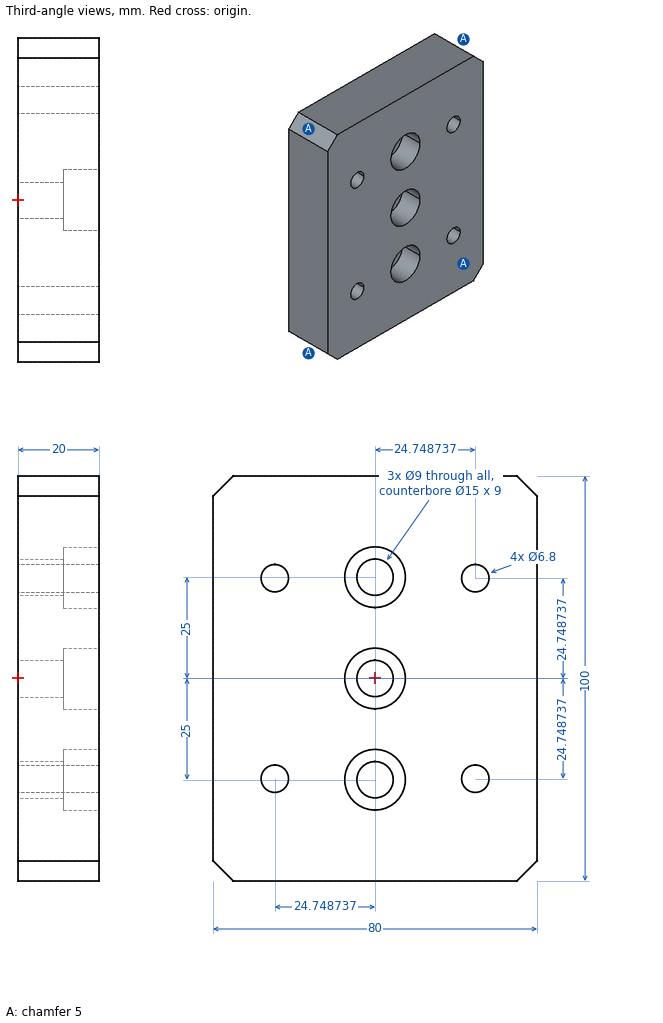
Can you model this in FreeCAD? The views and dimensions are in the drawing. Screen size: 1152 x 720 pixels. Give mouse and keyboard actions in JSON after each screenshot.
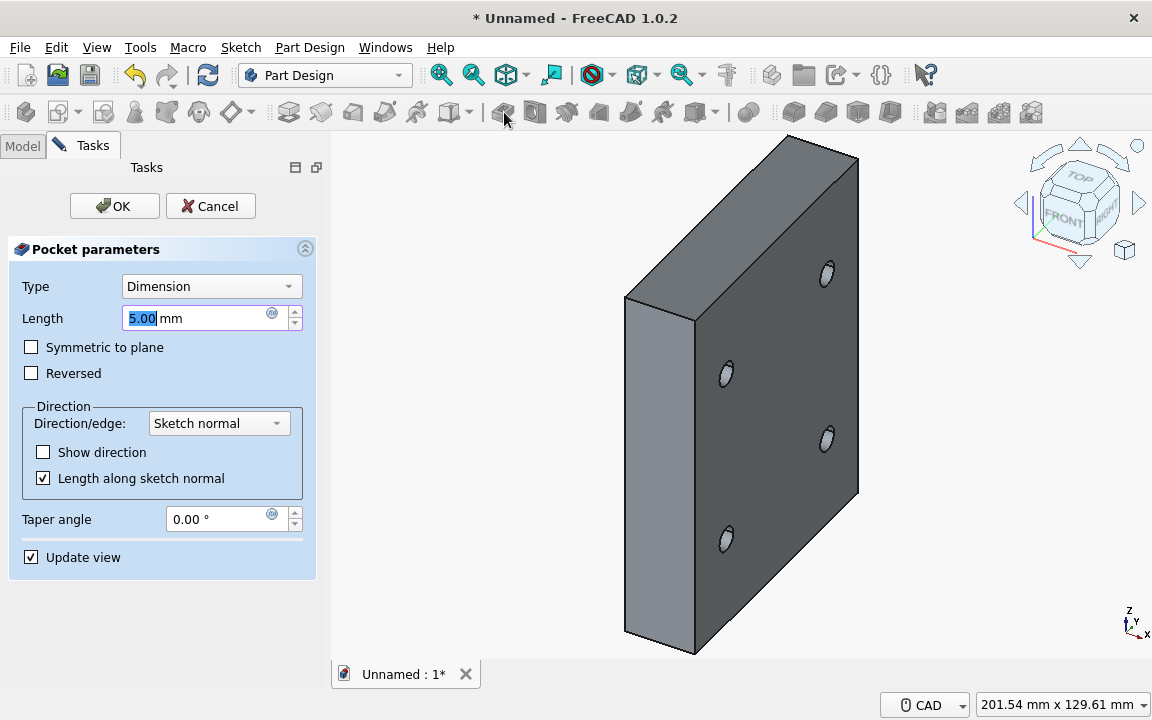
{"action": "left_click", "coordinate": [212, 286]}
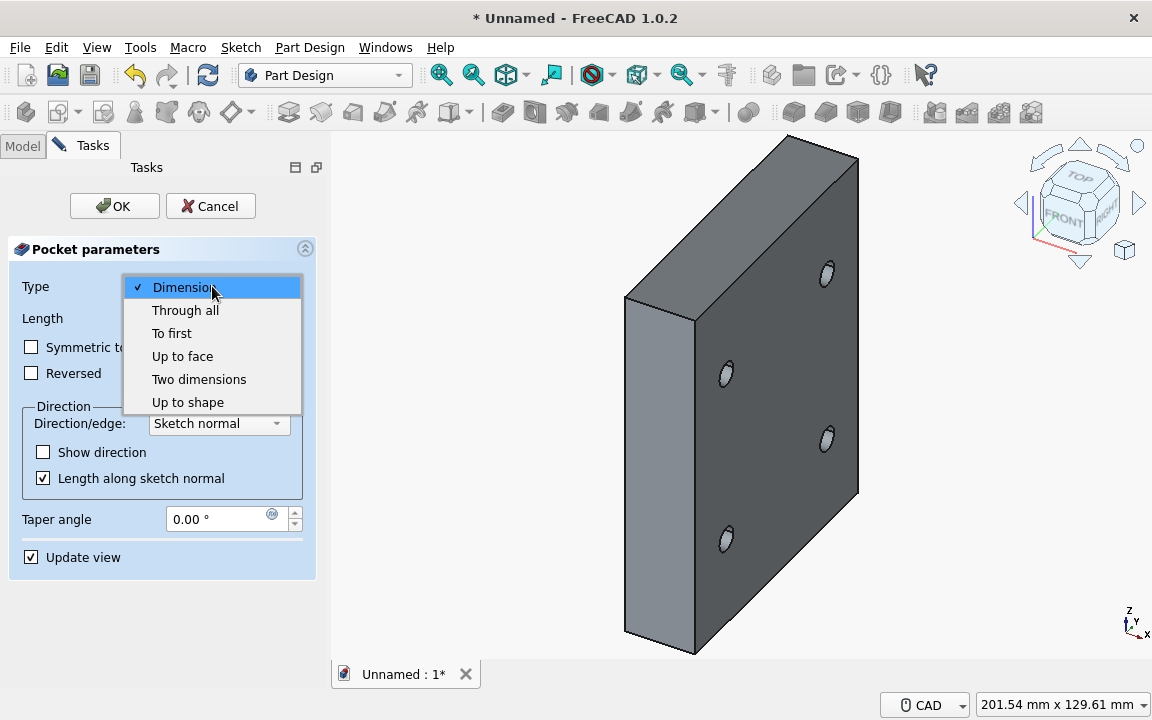
{"action": "left_click", "coordinate": [212, 310]}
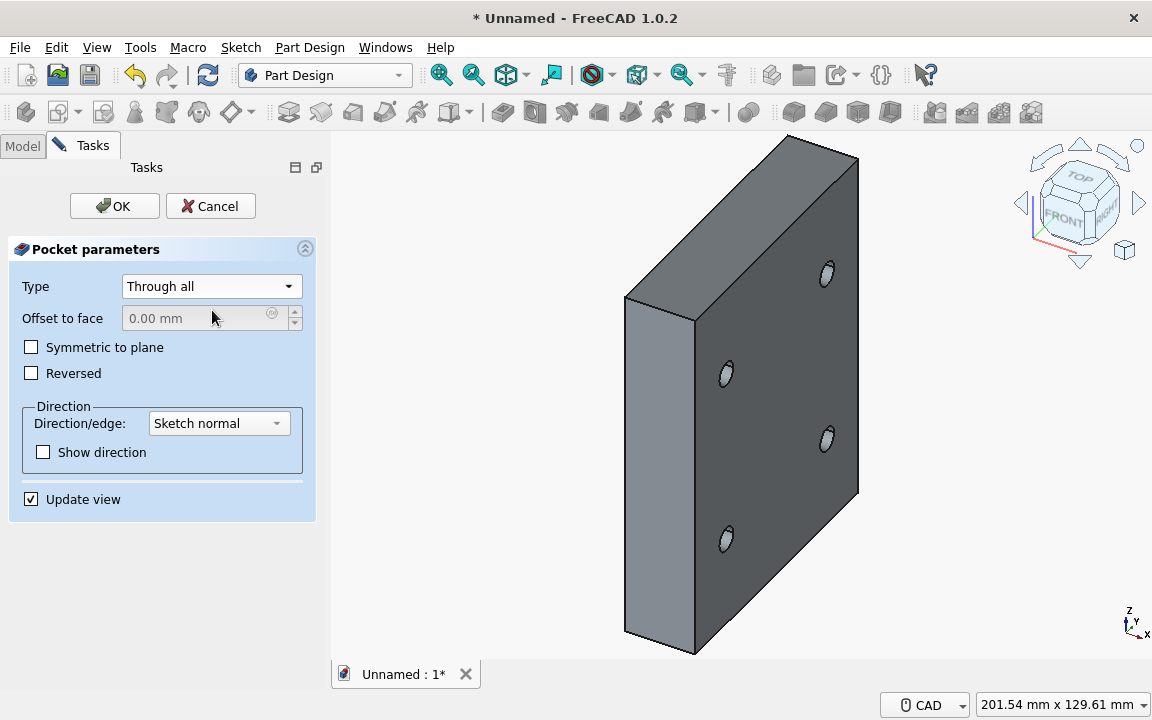
{"action": "left_click", "coordinate": [115, 206]}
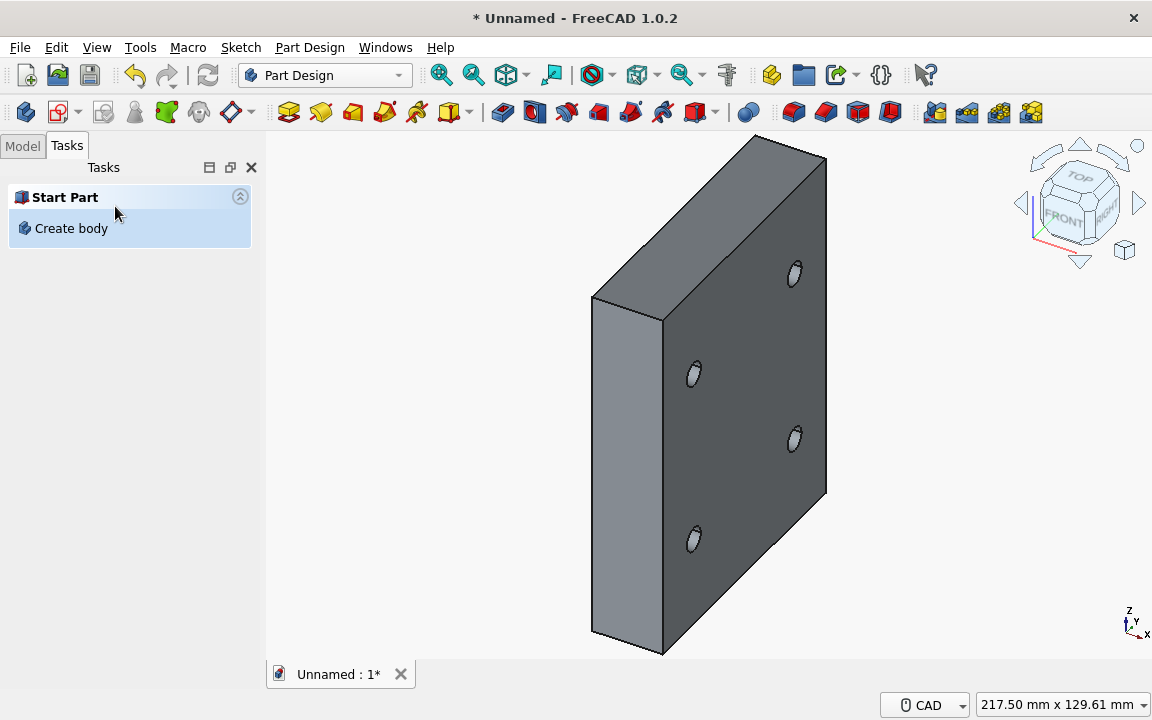
{"action": "left_click", "coordinate": [744, 406]}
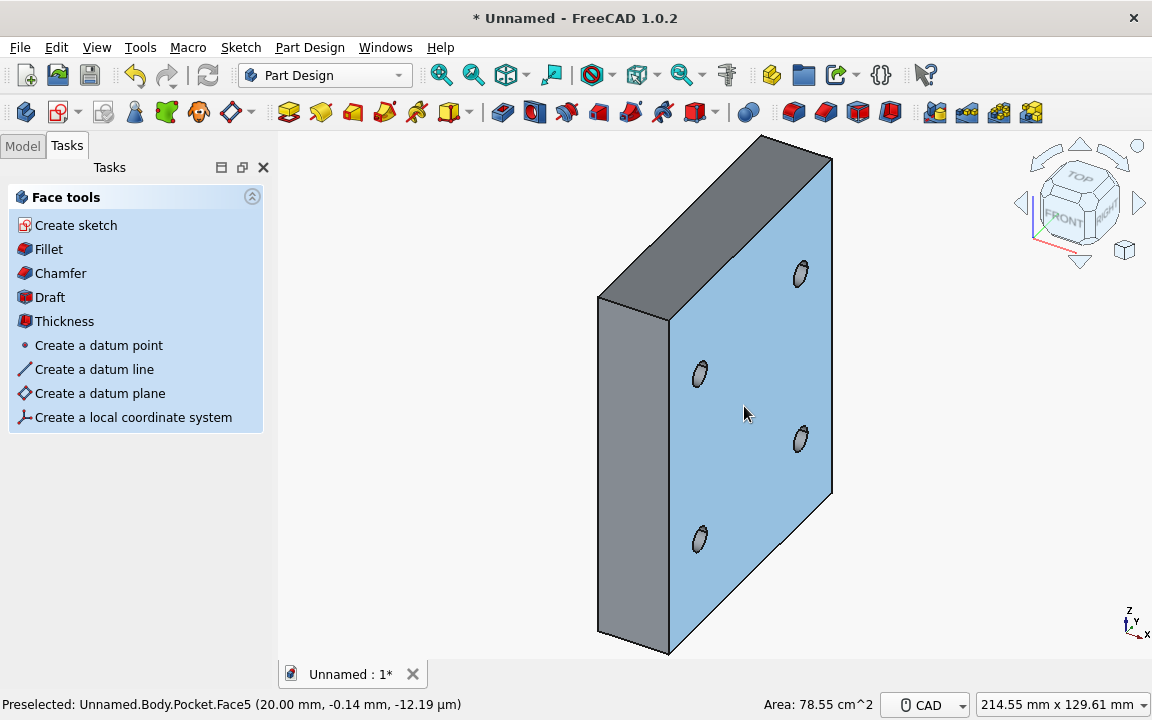
{"action": "left_click", "coordinate": [58, 112]}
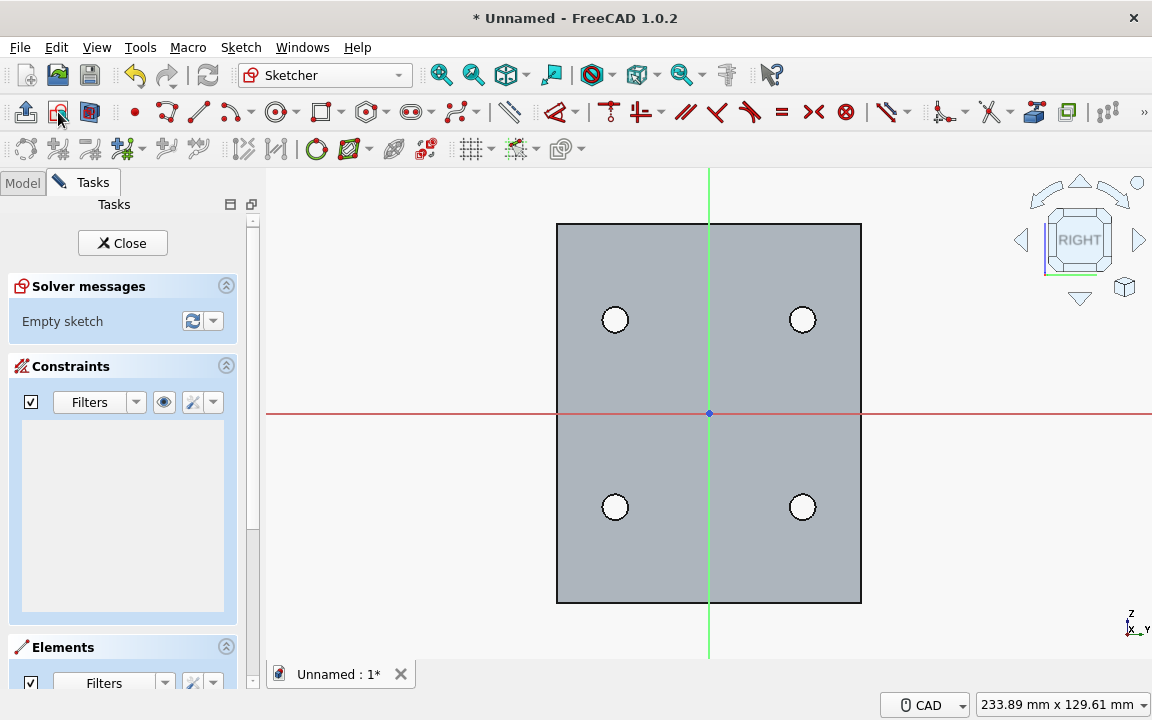
{"action": "scroll", "coordinate": [848, 413], "scroll_direction": "up", "scroll_amount": 2}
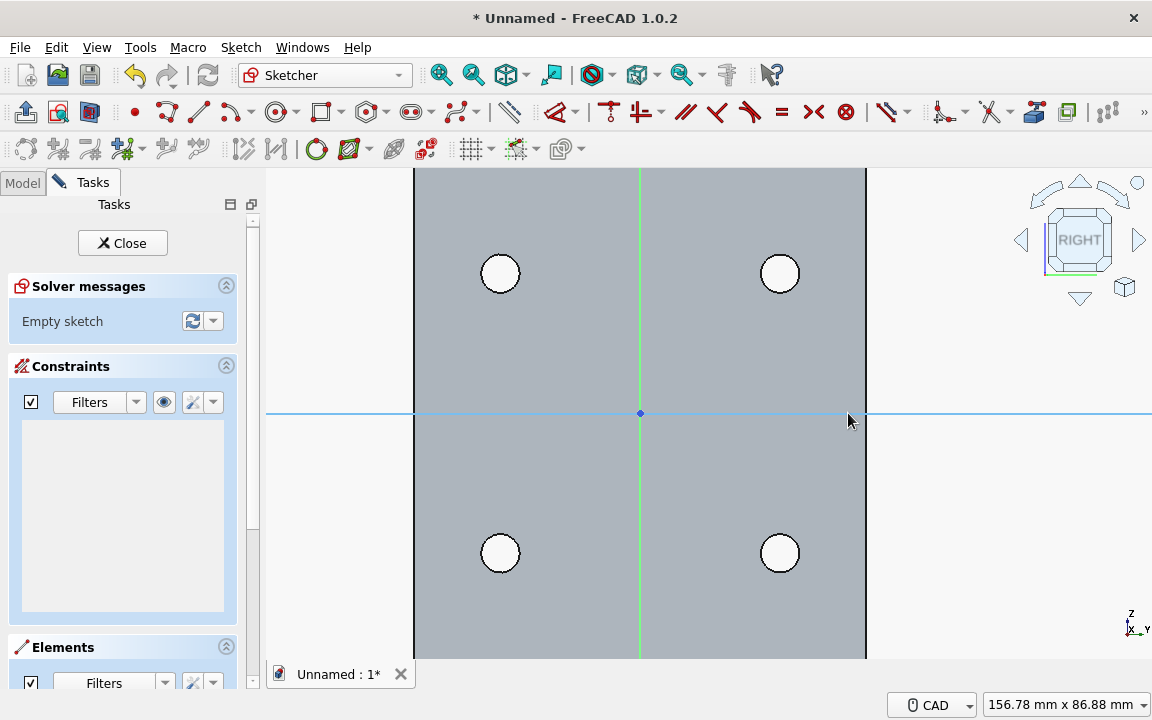
{"action": "key", "text": "g c"}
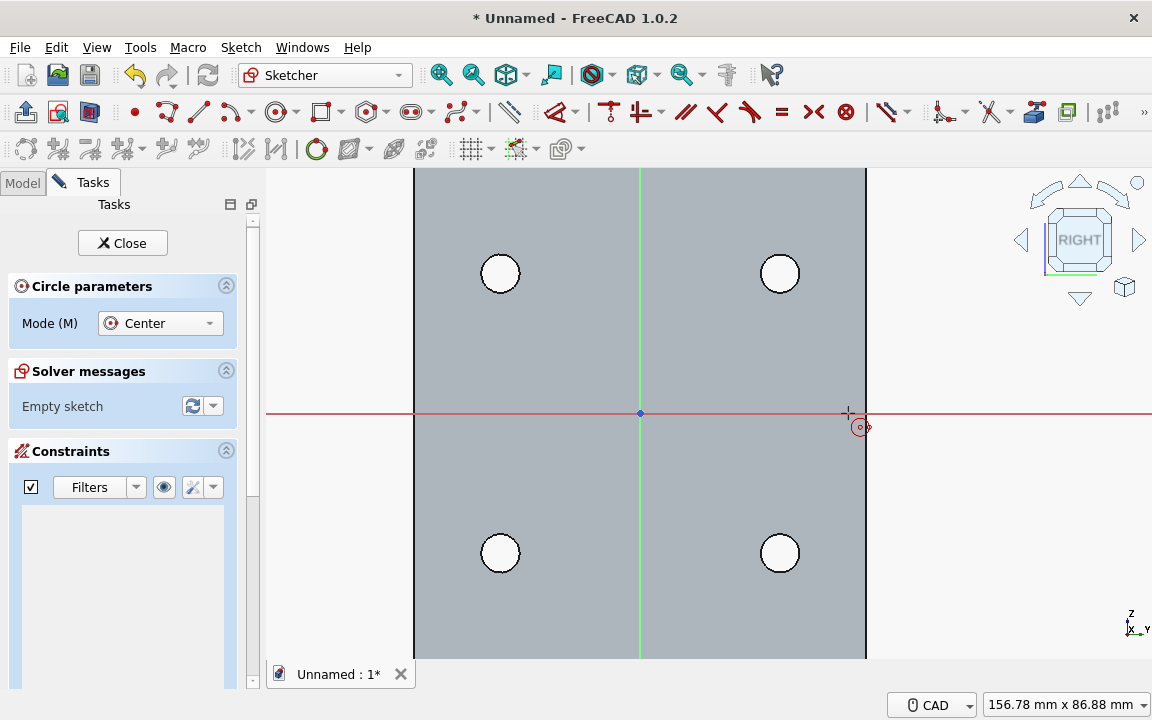
{"action": "left_click", "coordinate": [640, 272]}
{"action": "mouse_move", "coordinate": [658, 254]}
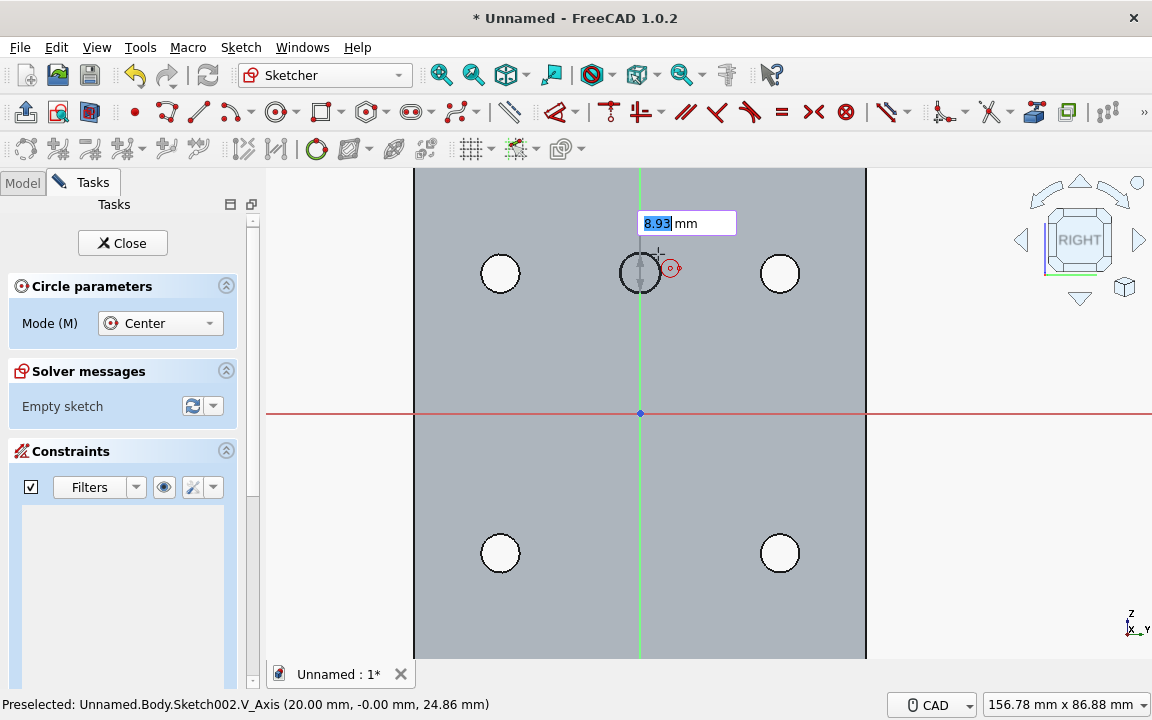
{"action": "type", "text": "9"}
{"action": "key", "text": "Return"}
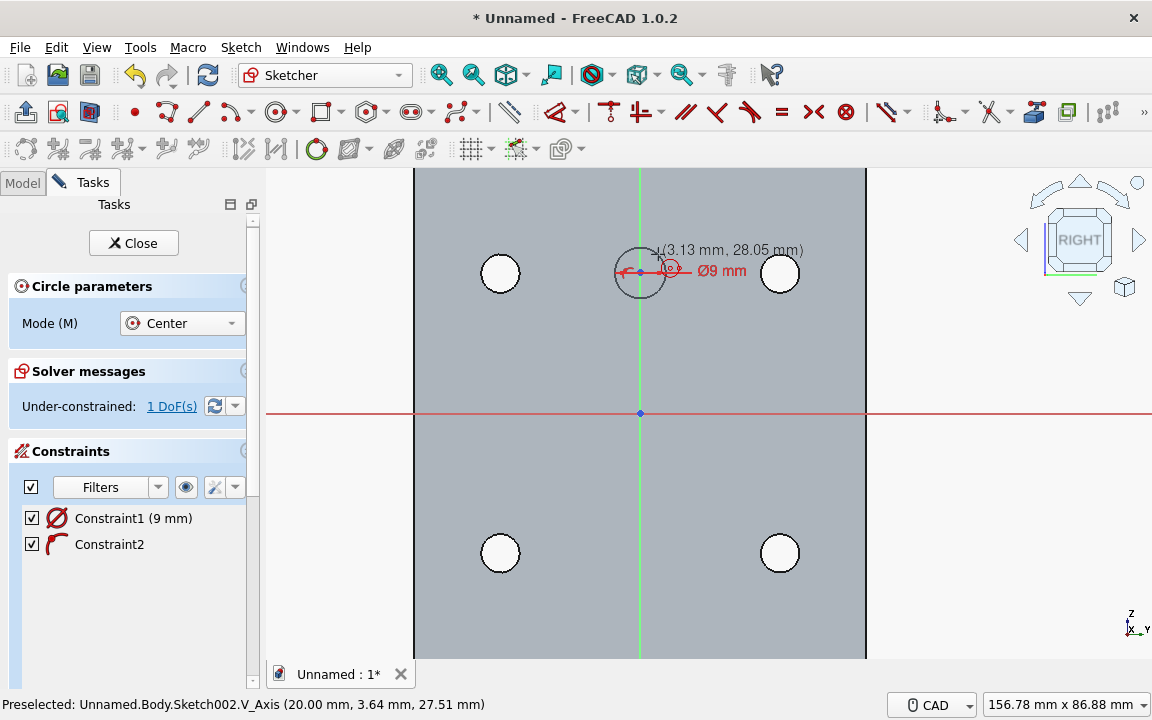
{"action": "left_click", "coordinate": [640, 414]}
{"action": "mouse_move", "coordinate": [658, 396]}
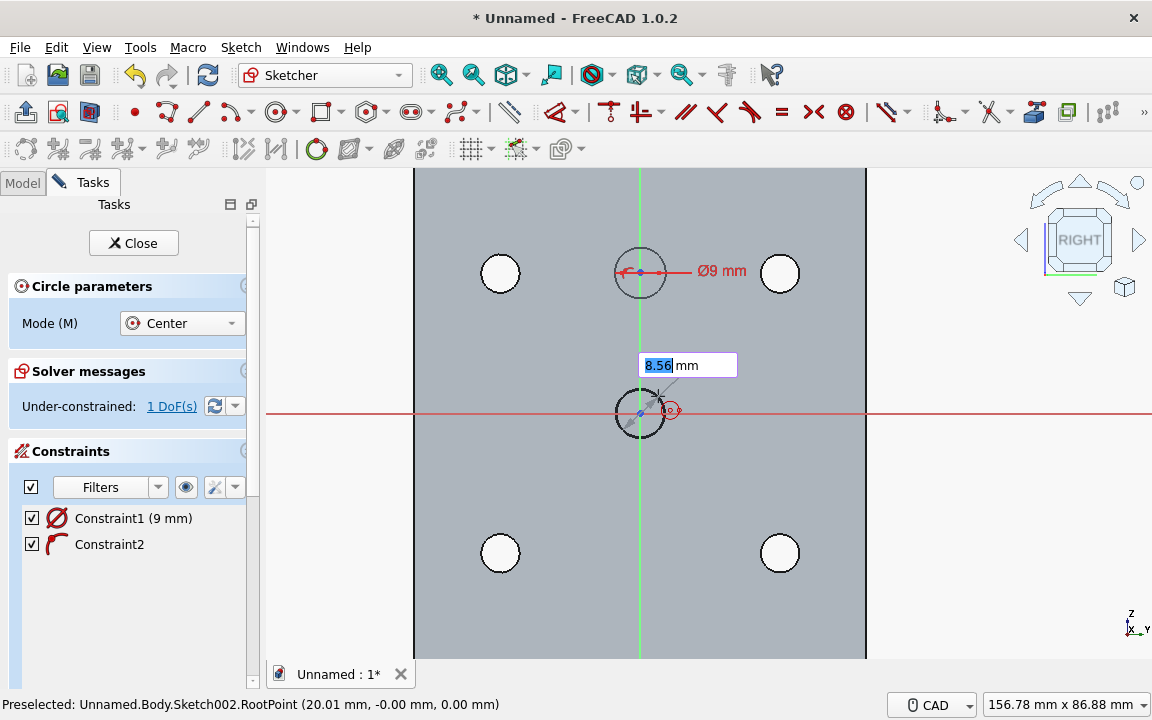
{"action": "type", "text": "9"}
{"action": "key", "text": "Return"}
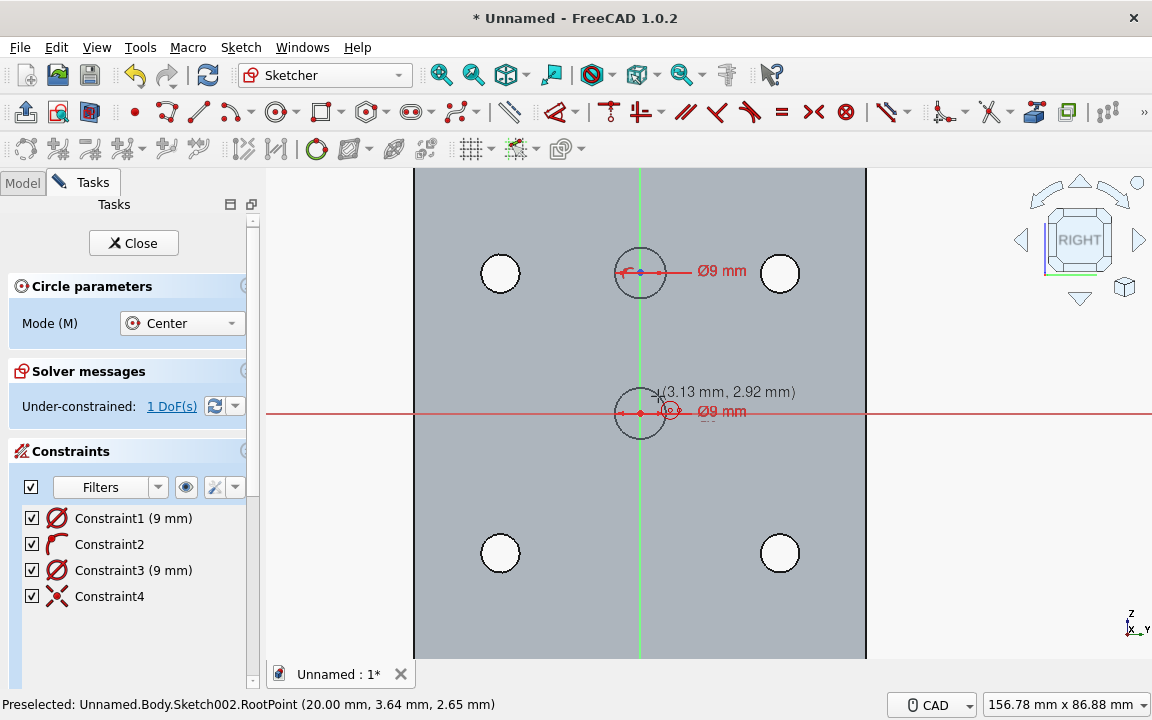
{"action": "left_click", "coordinate": [640, 555]}
{"action": "mouse_move", "coordinate": [658, 537]}